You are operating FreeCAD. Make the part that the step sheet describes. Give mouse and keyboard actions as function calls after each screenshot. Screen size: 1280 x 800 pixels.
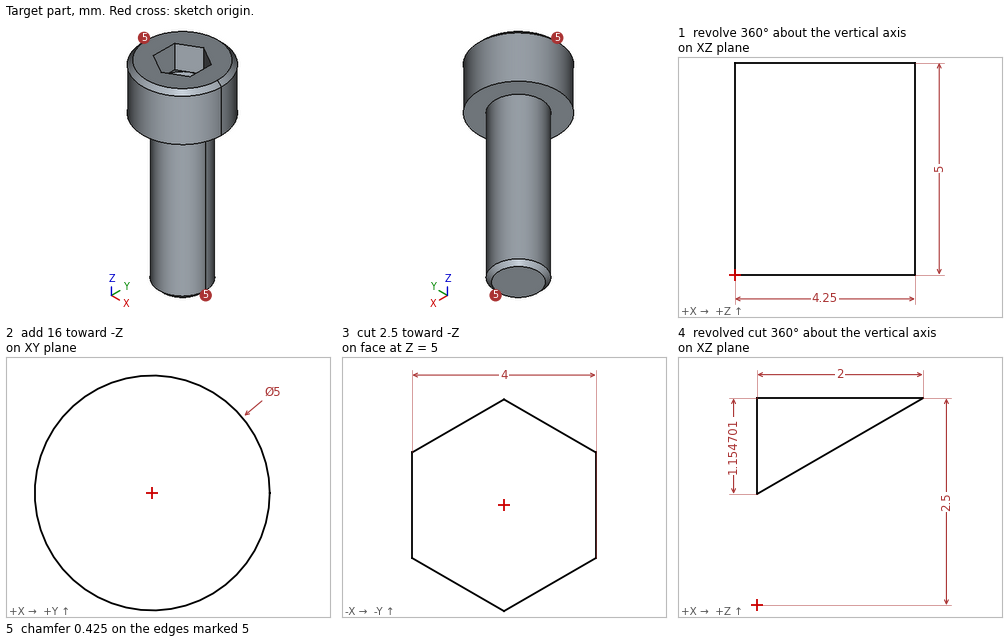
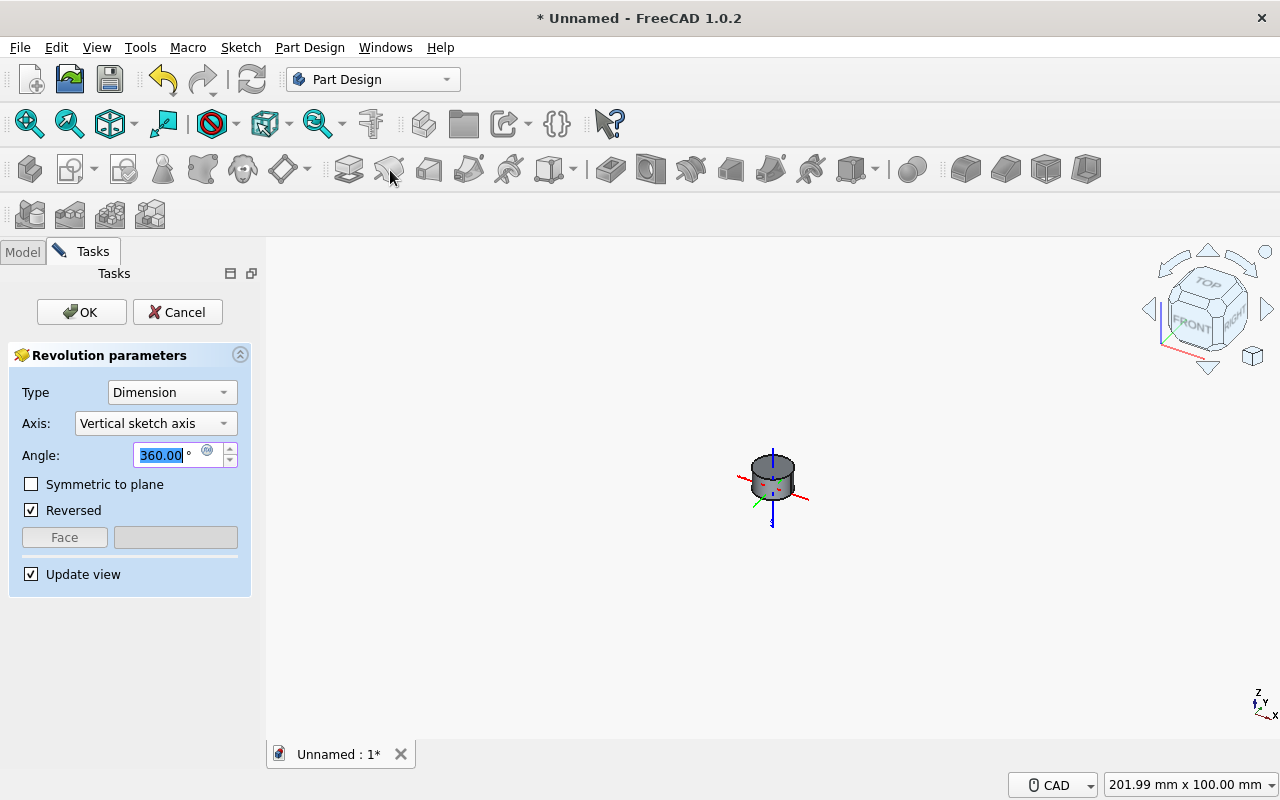
click(82, 312)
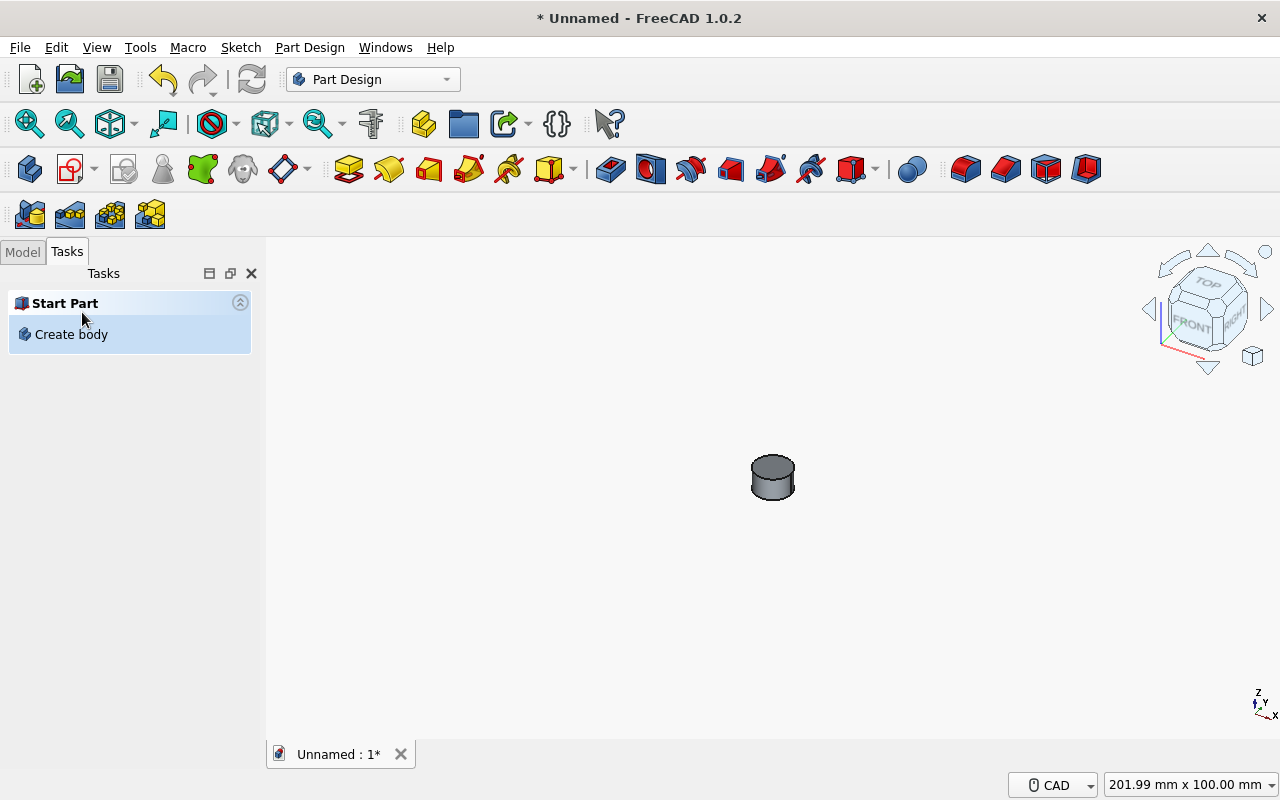
click(30, 124)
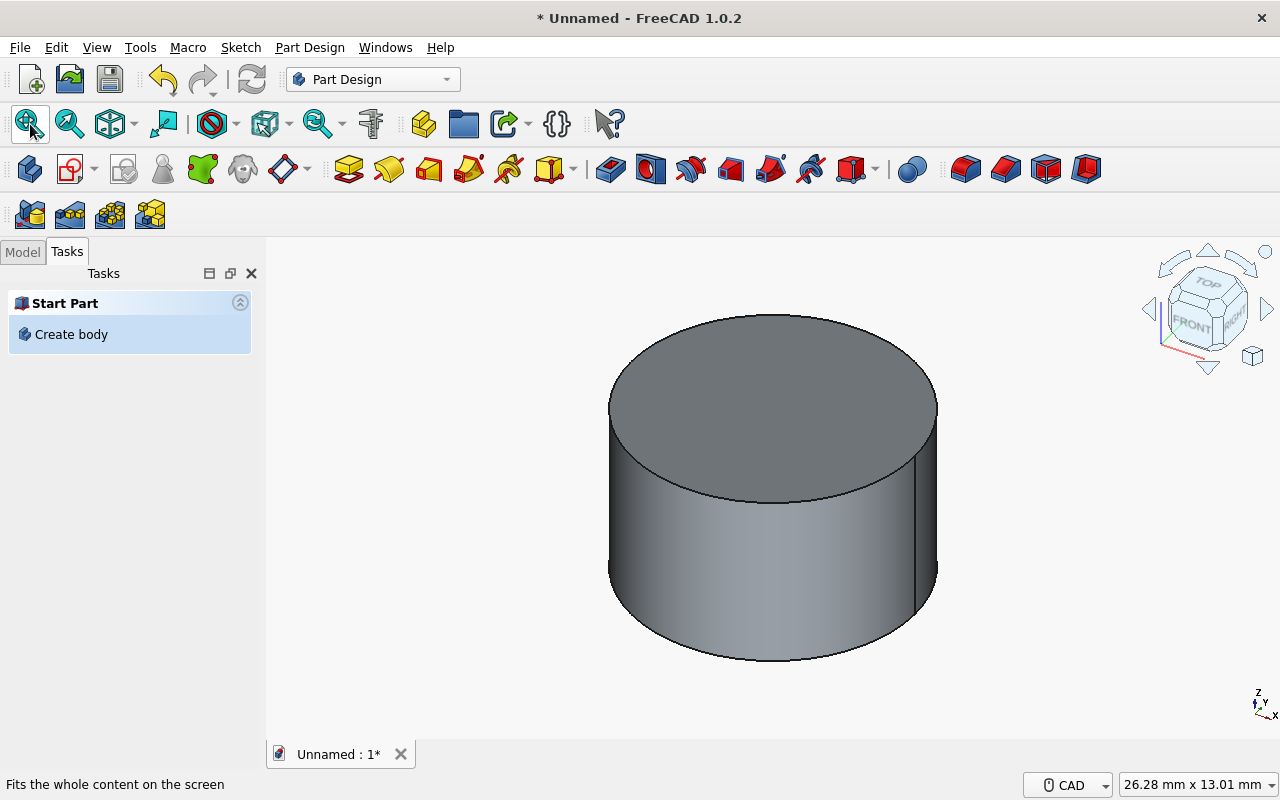
click(70, 170)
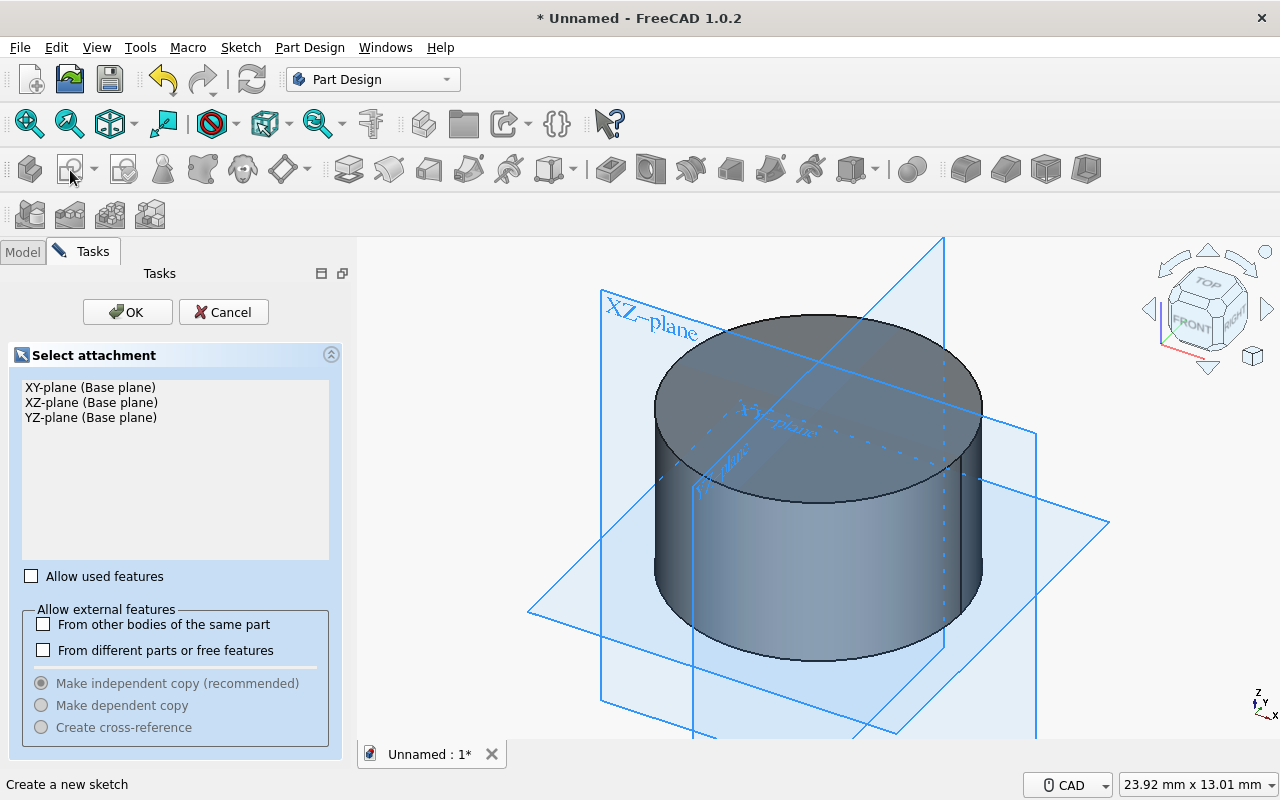
click(82, 388)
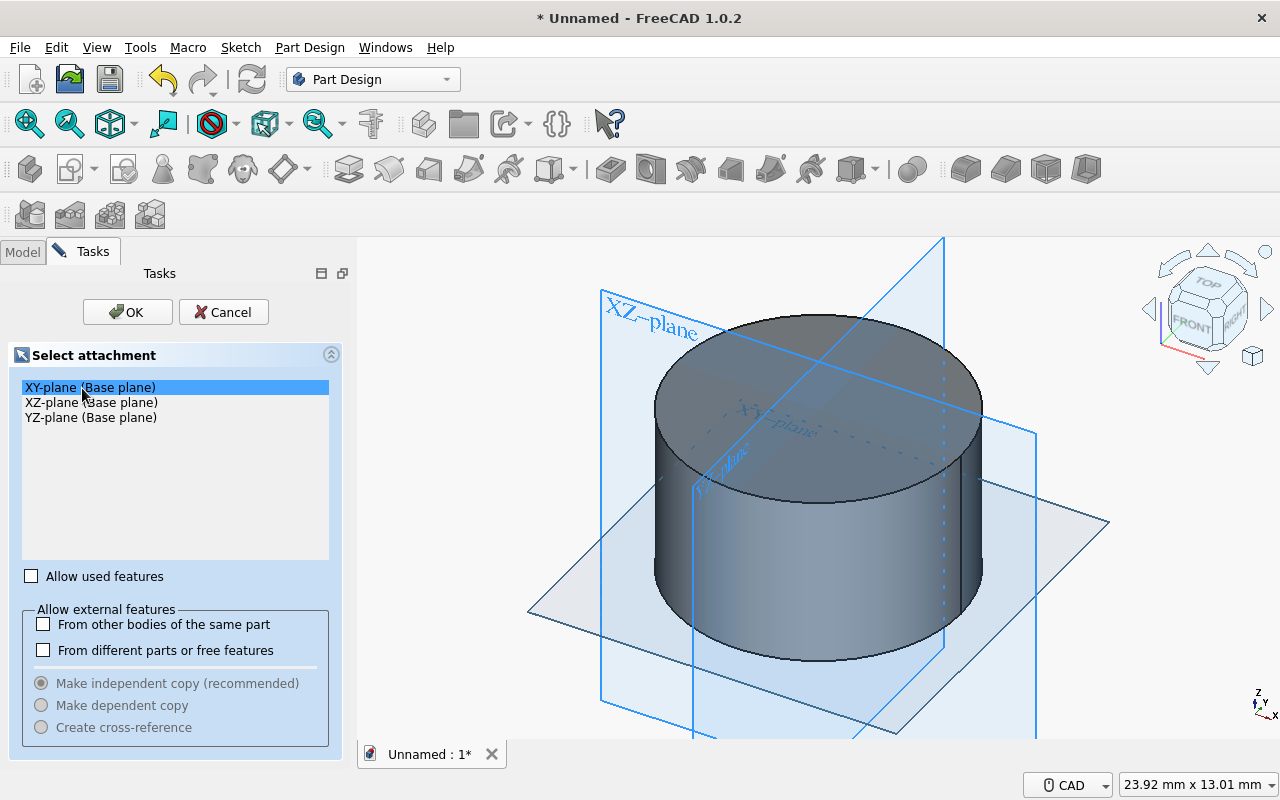
click(128, 312)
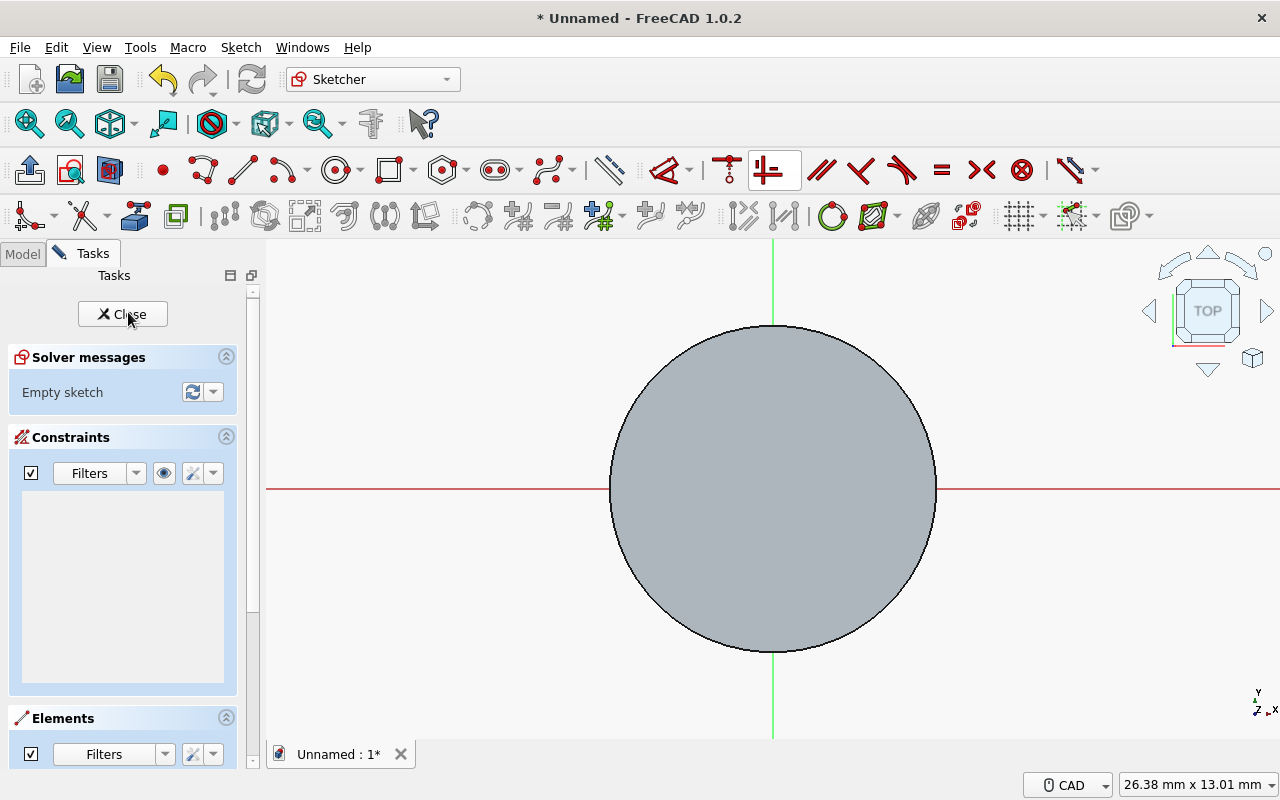
click(110, 170)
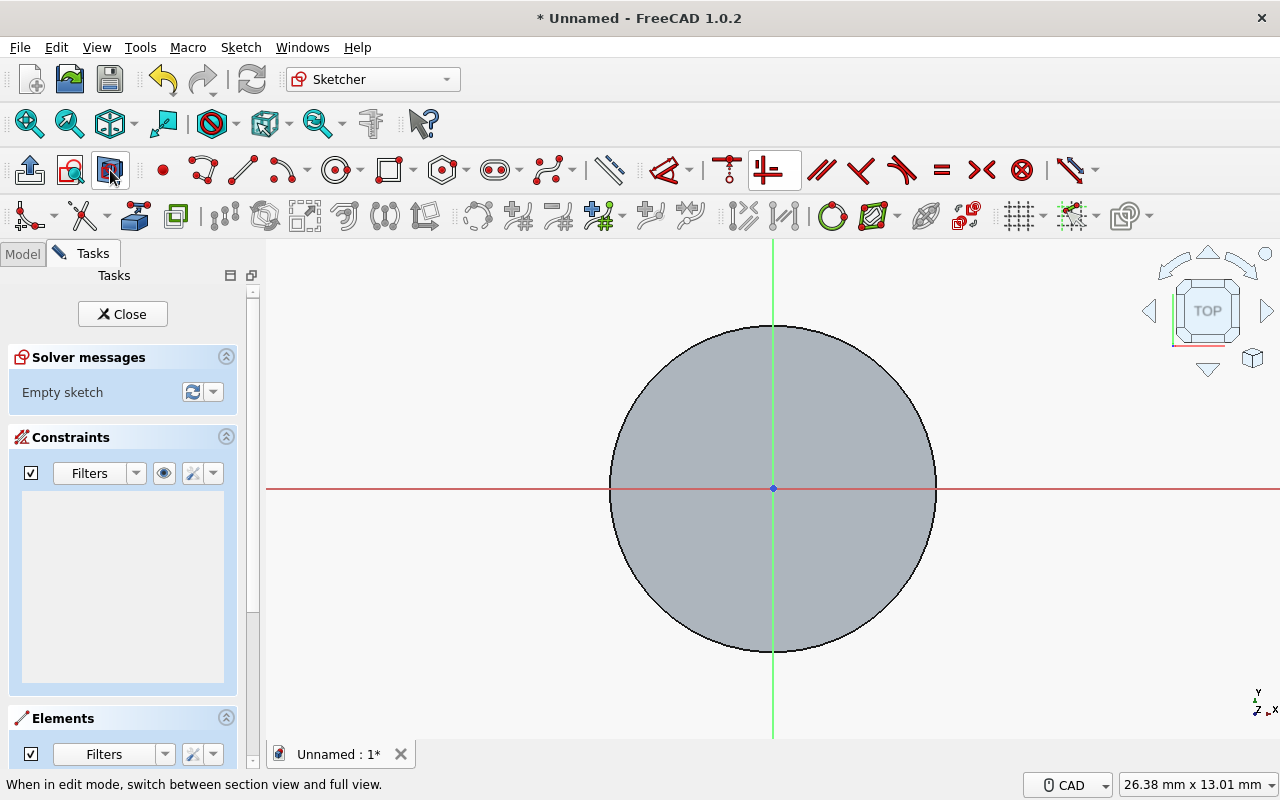
scroll(912, 489, up, 2)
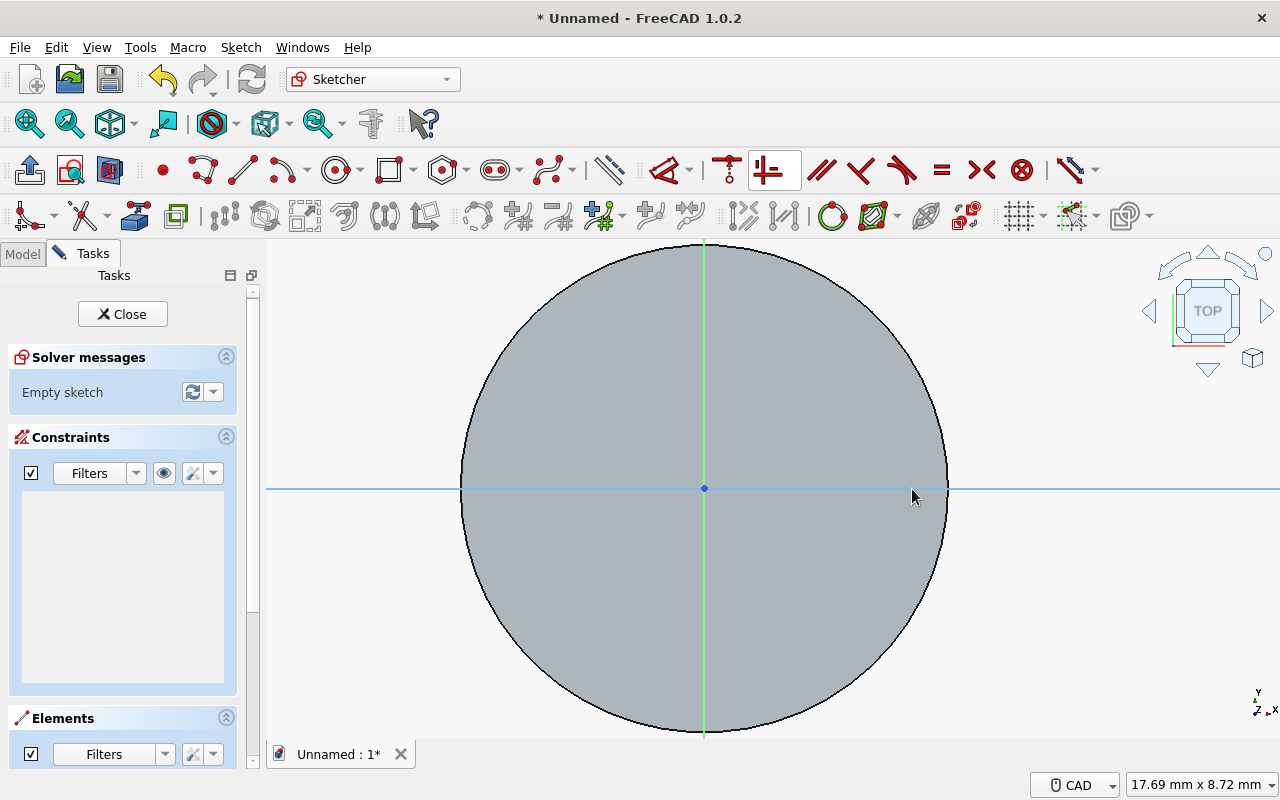
click(336, 170)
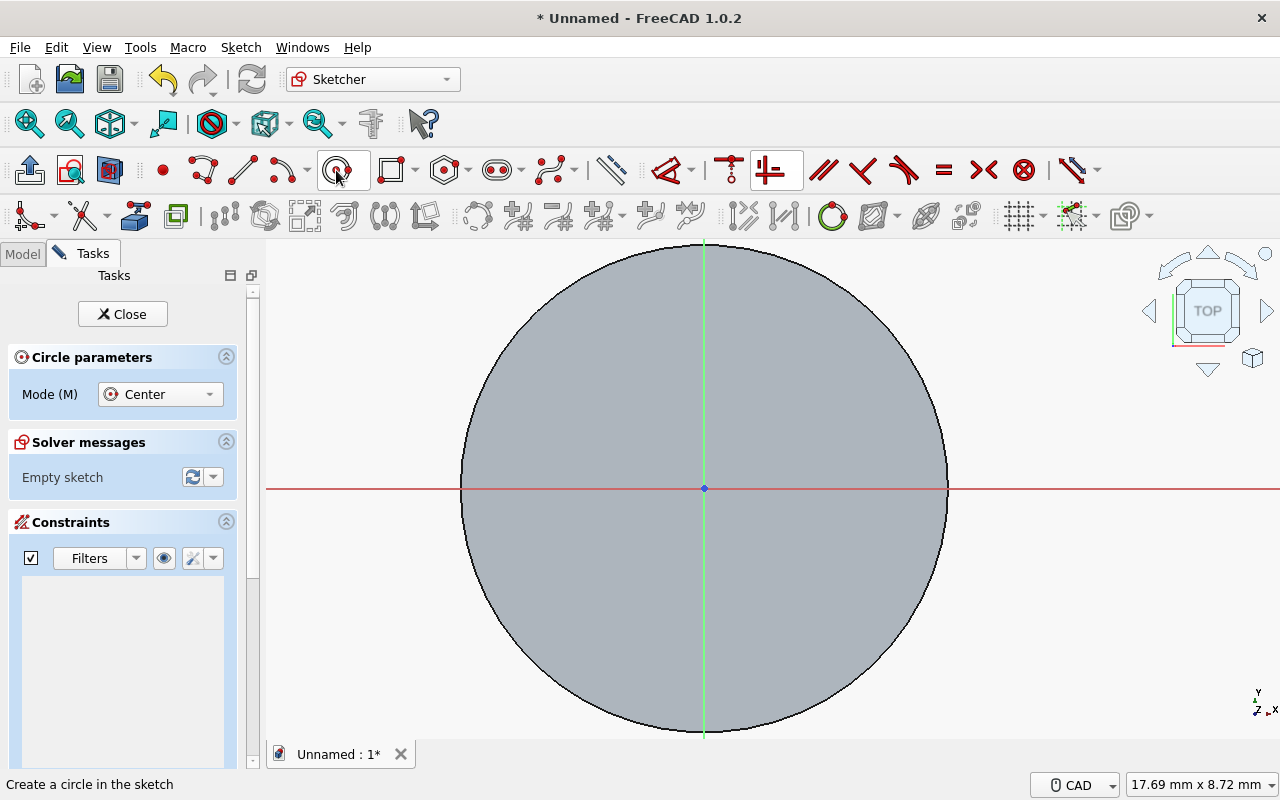
click(704, 489)
move(806, 387)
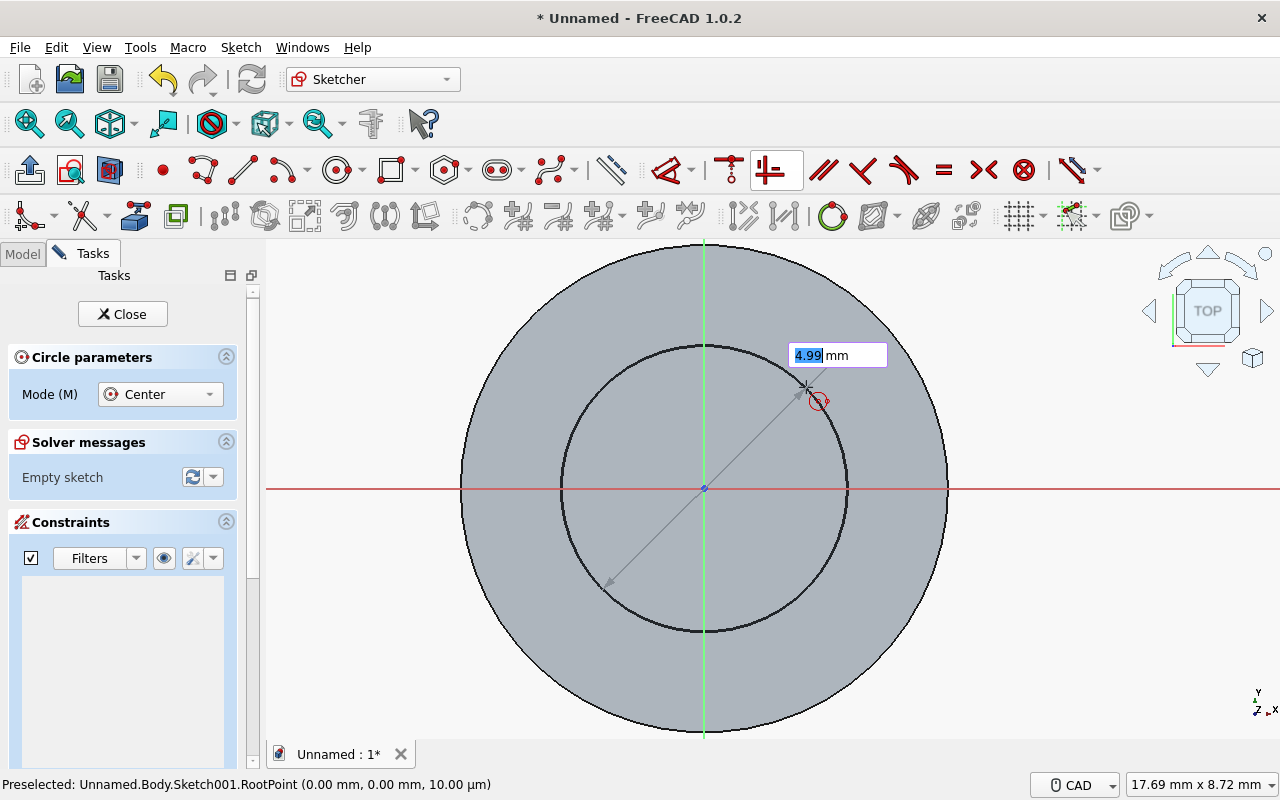
text(5)
key(Return)
key(Escape)